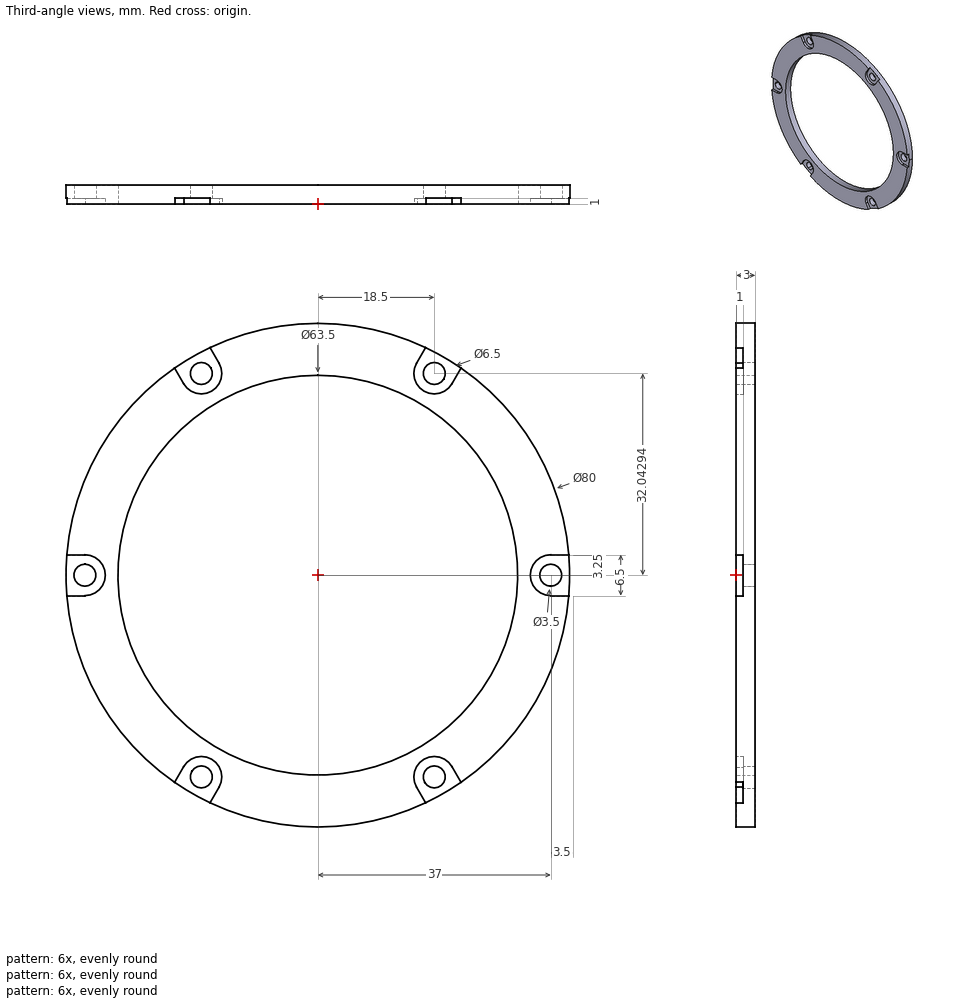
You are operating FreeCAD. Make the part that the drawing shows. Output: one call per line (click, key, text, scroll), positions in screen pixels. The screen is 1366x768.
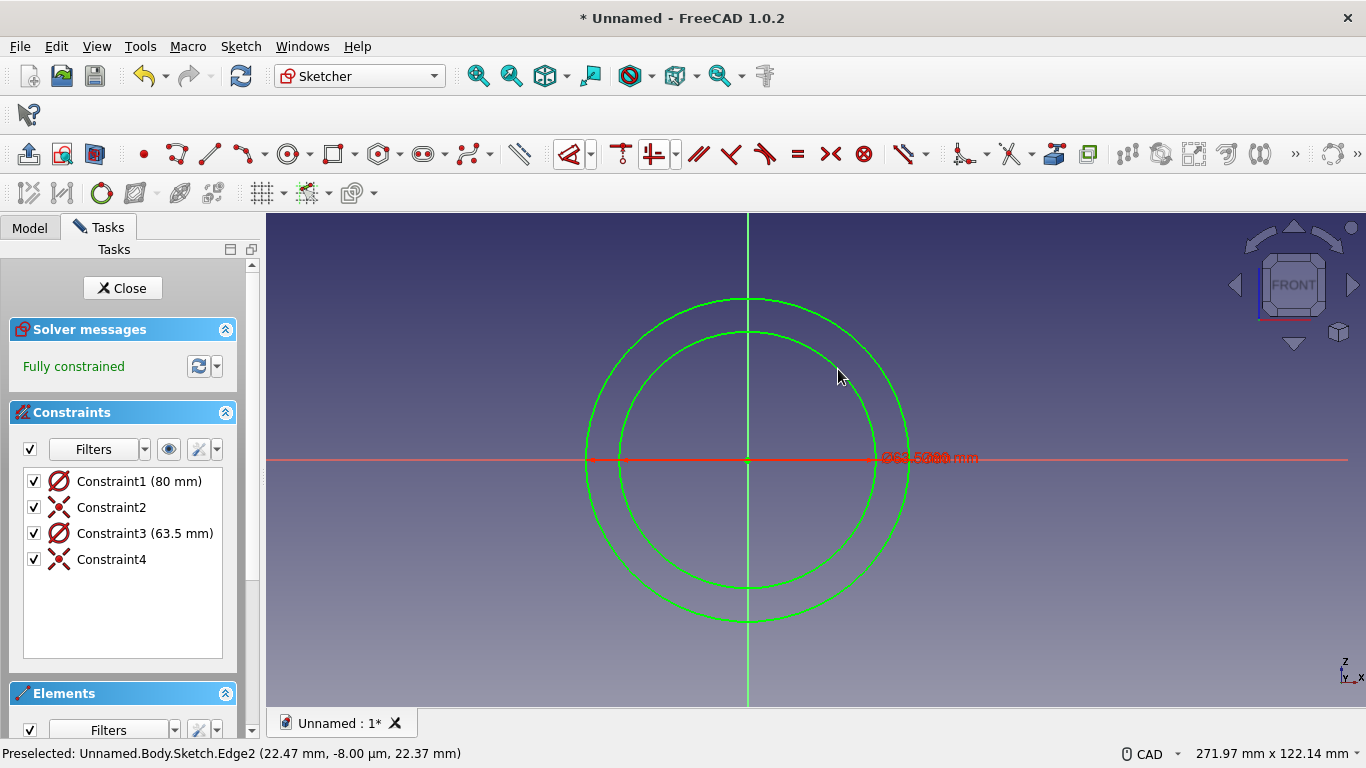
click(123, 288)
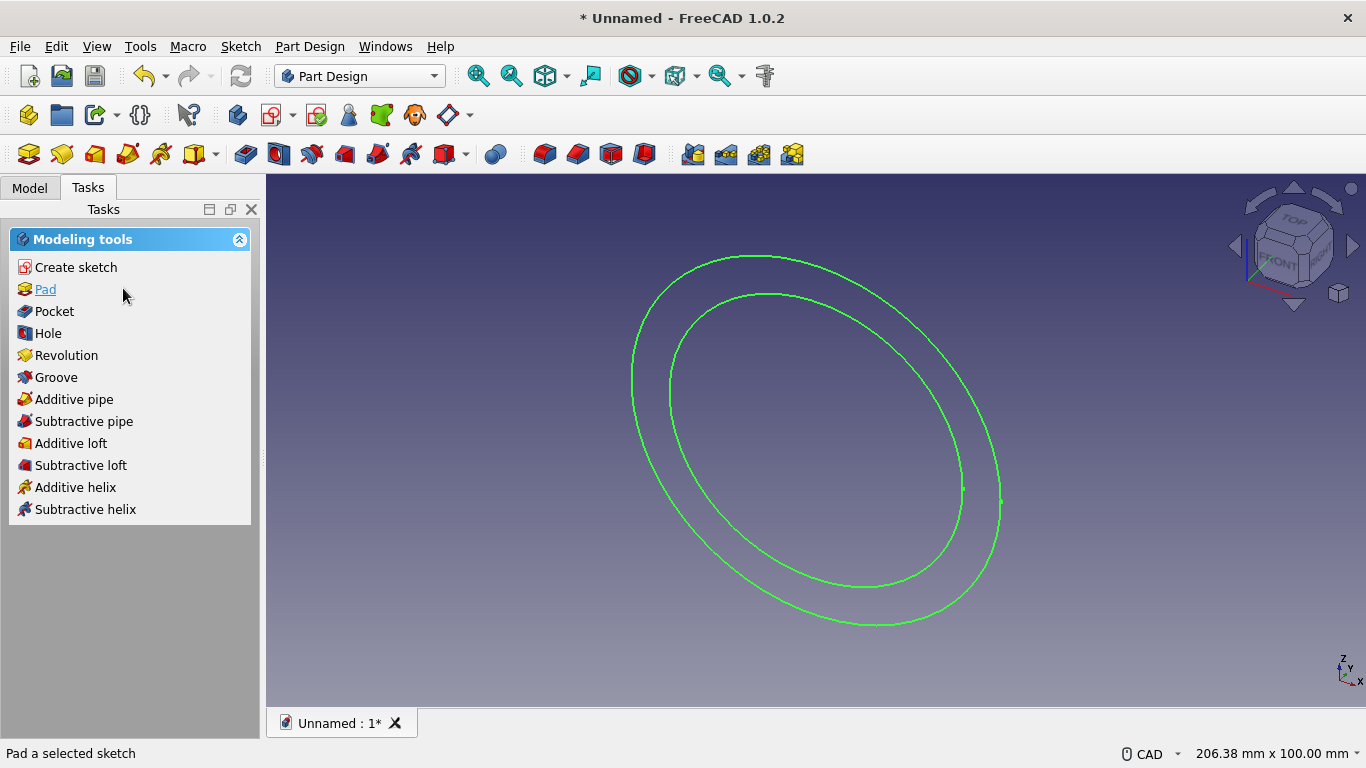
click(29, 154)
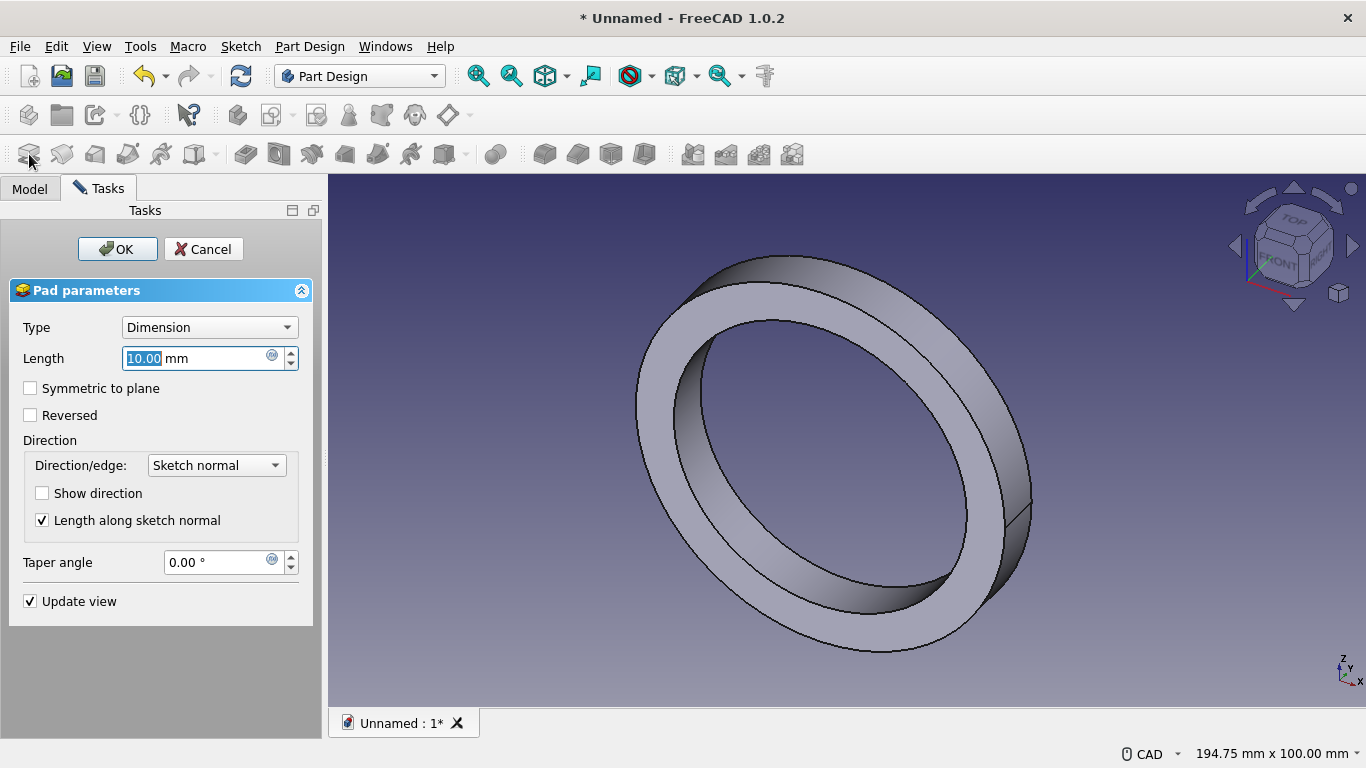
text(3)
key(Tab)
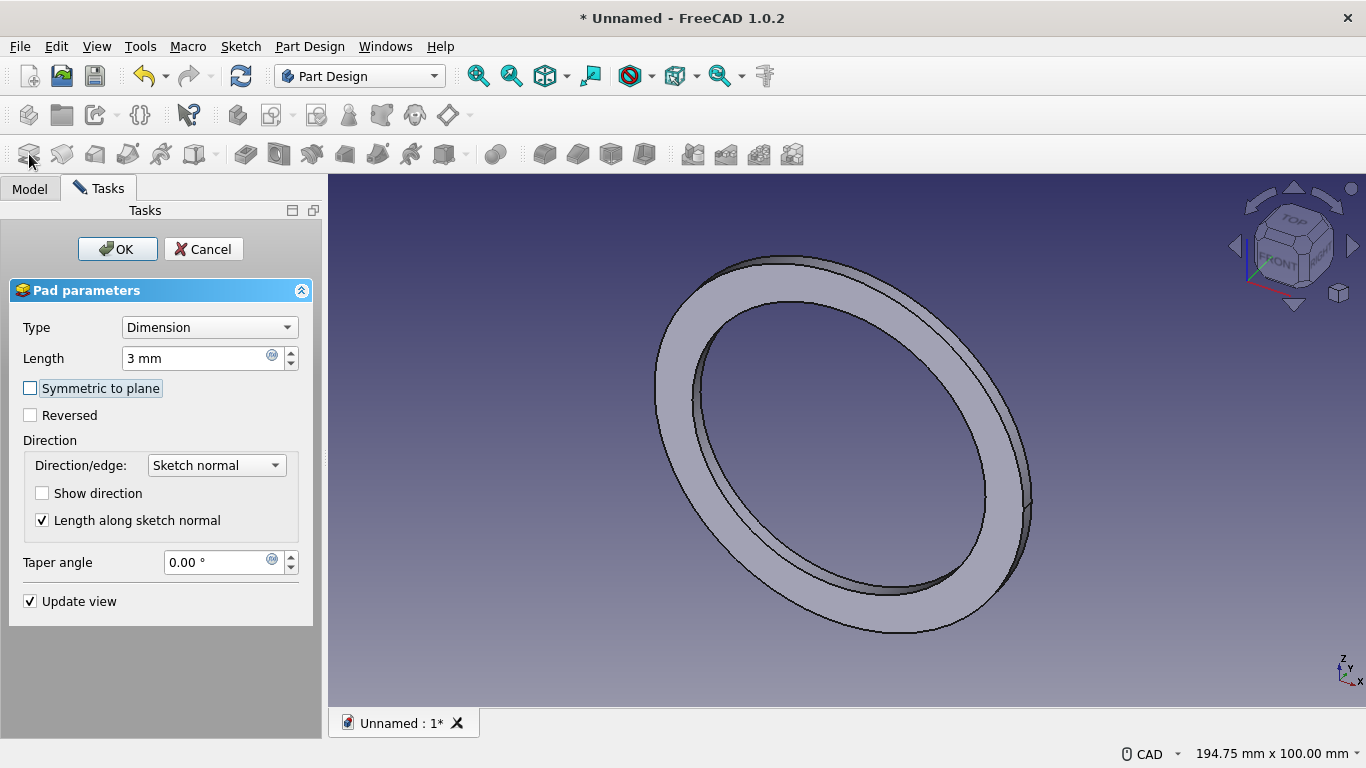
click(31, 415)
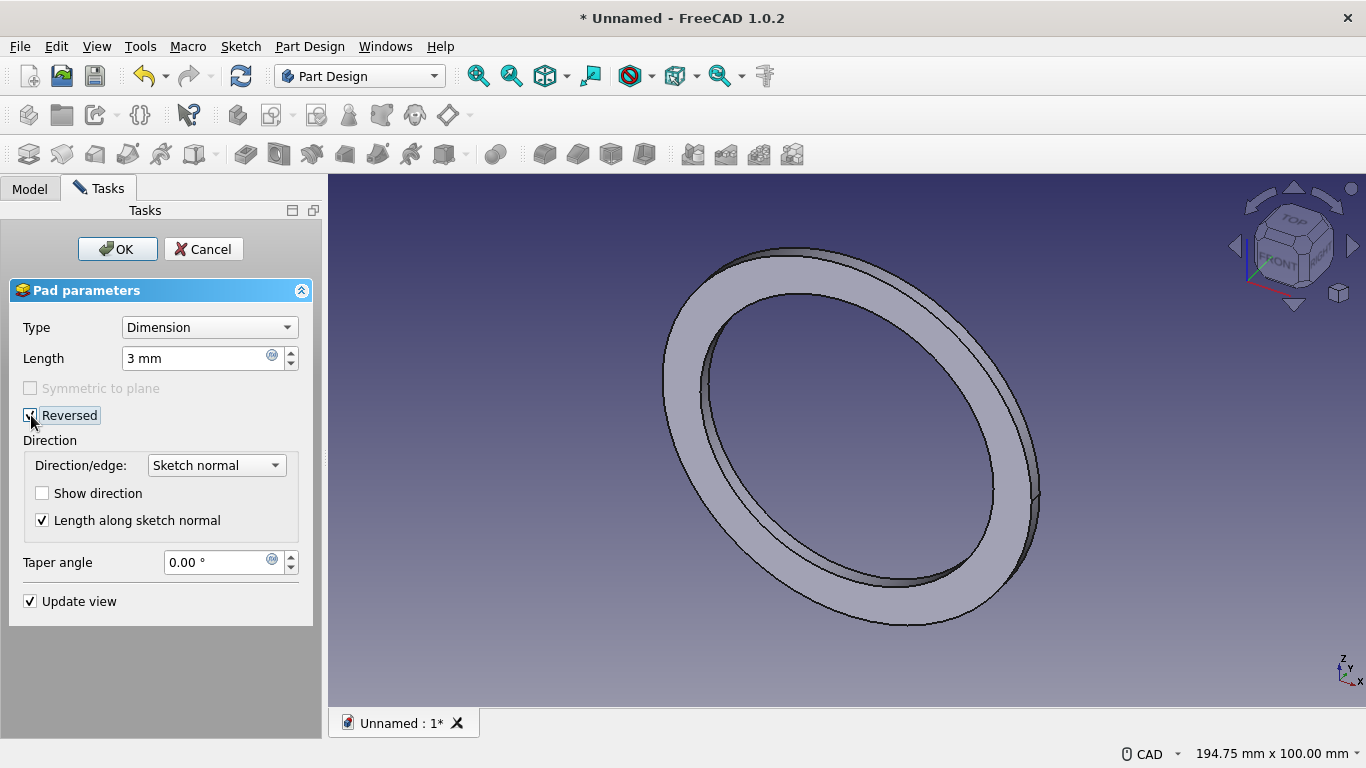
click(118, 249)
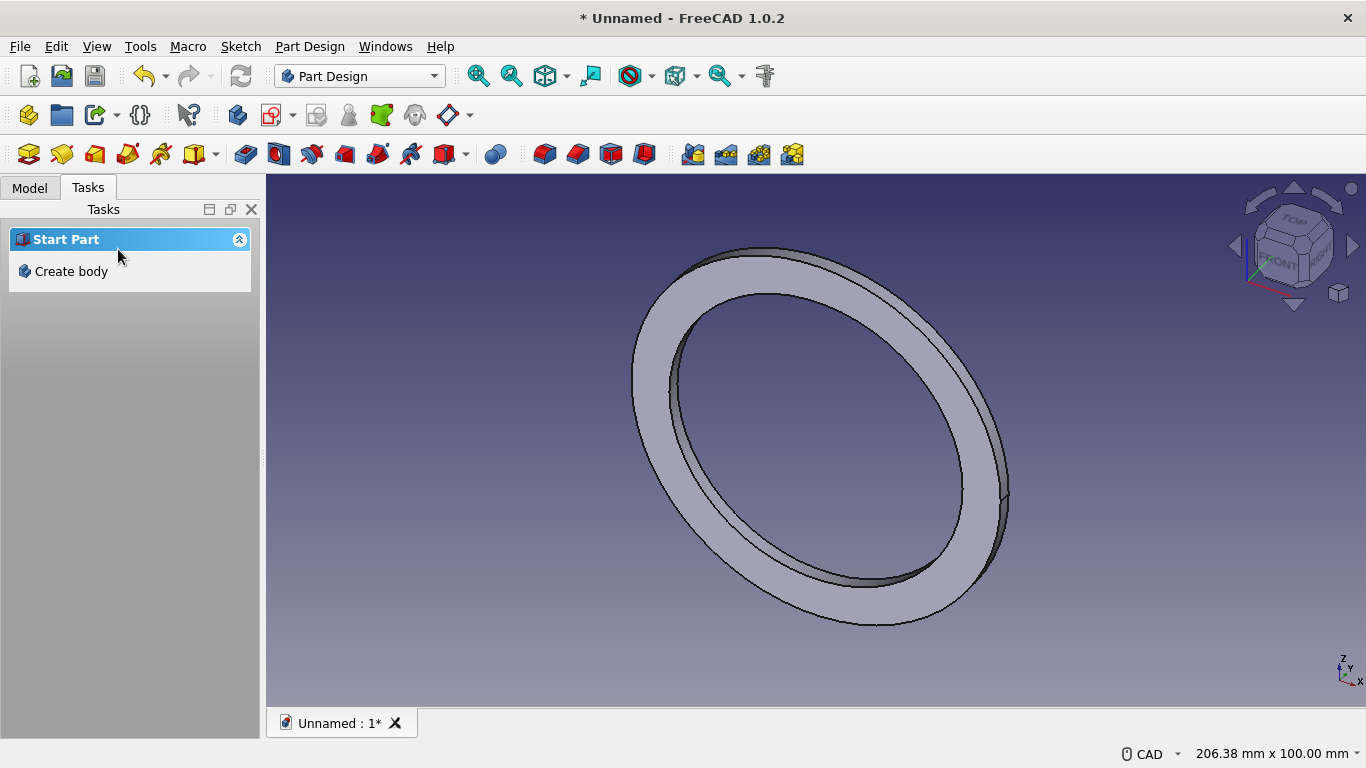
click(763, 572)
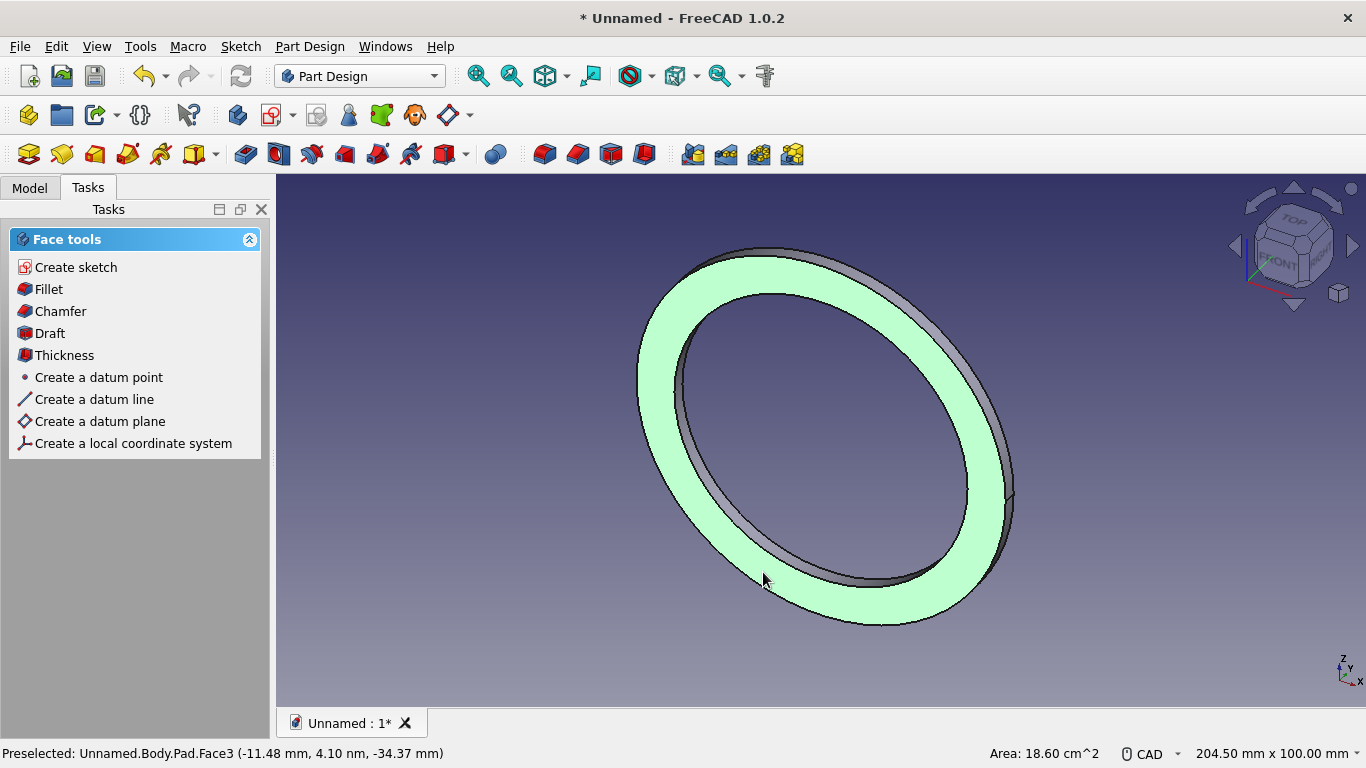
click(270, 116)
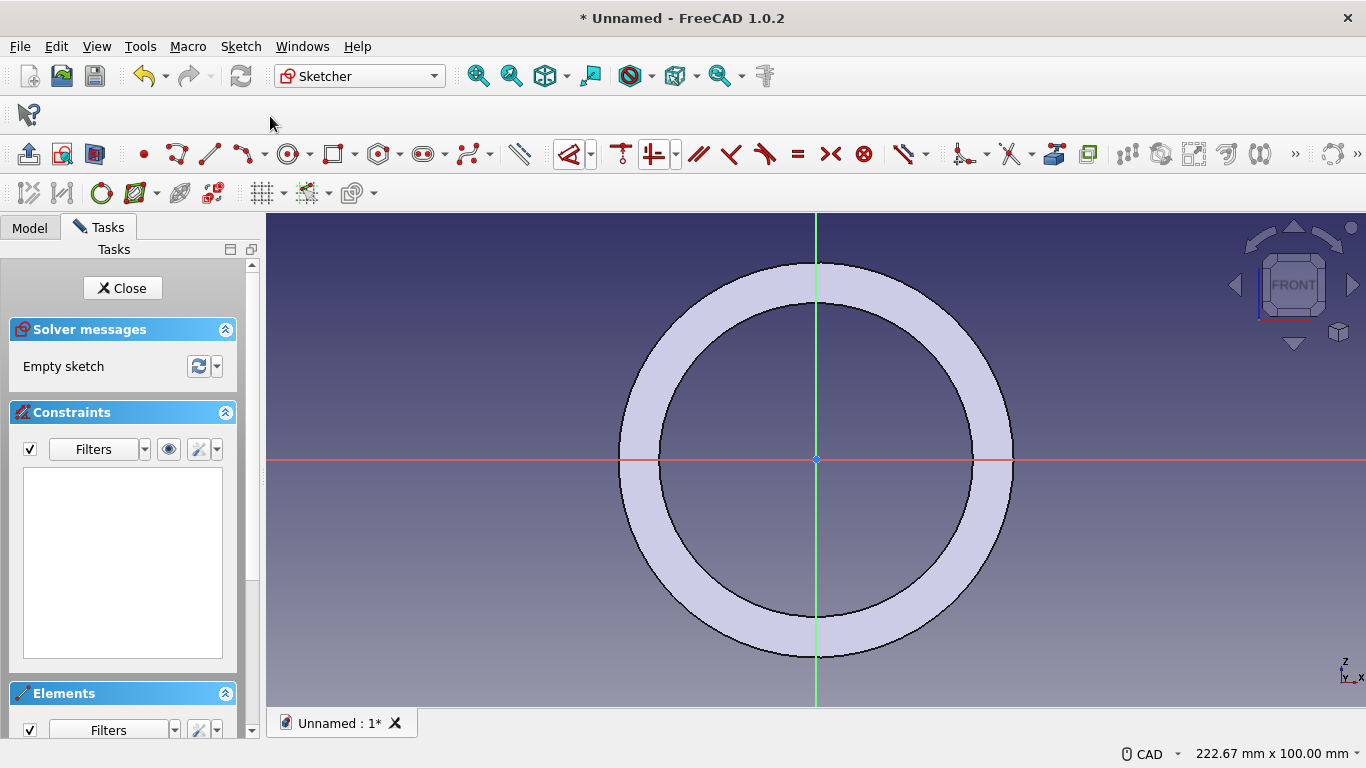
scroll(1015, 460, up, 14)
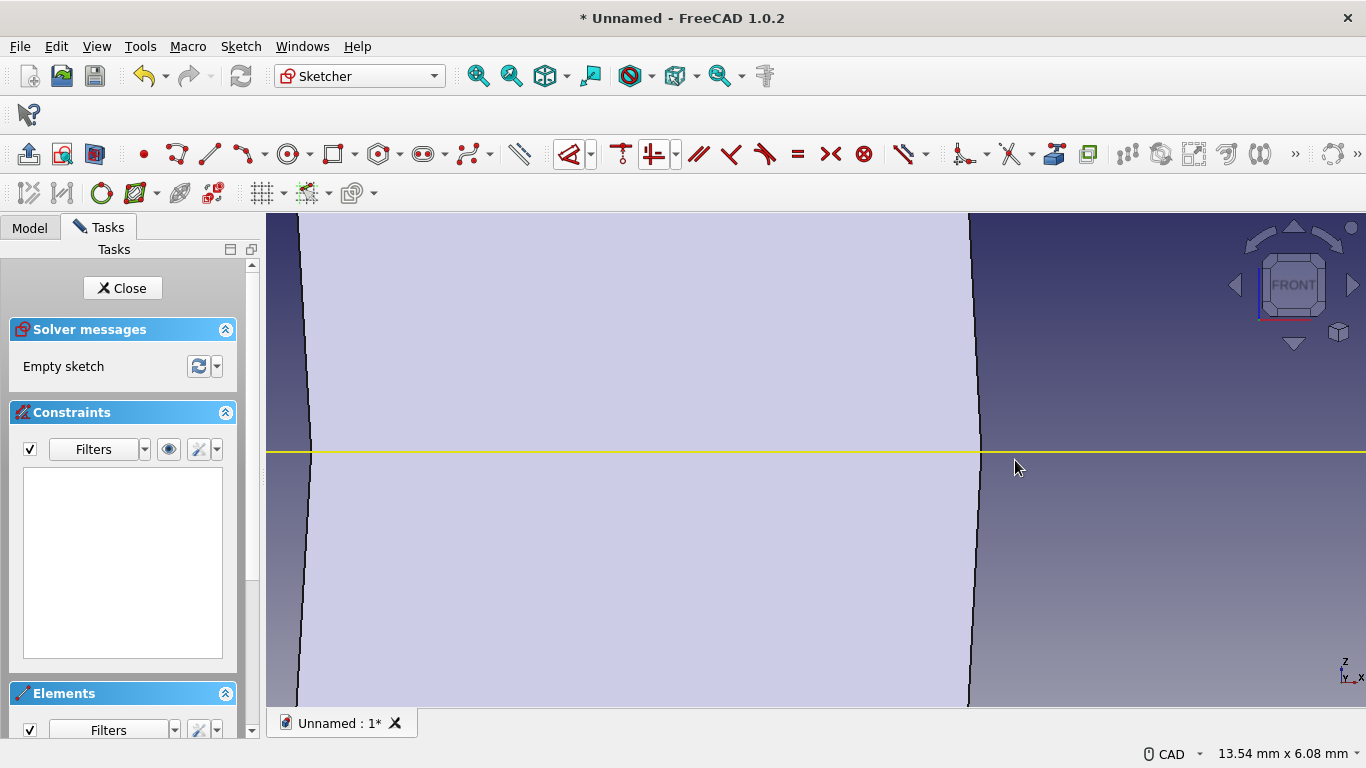
click(288, 154)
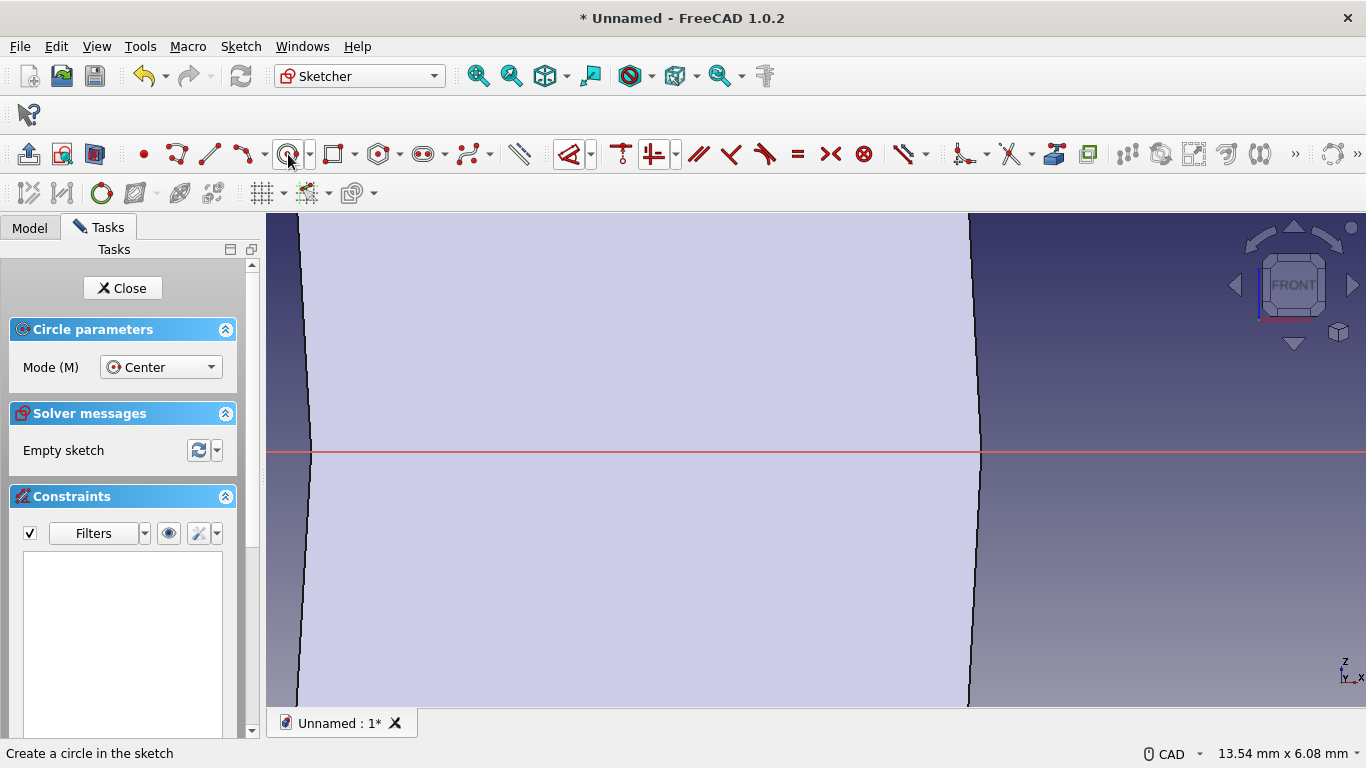
click(738, 452)
move(838, 352)